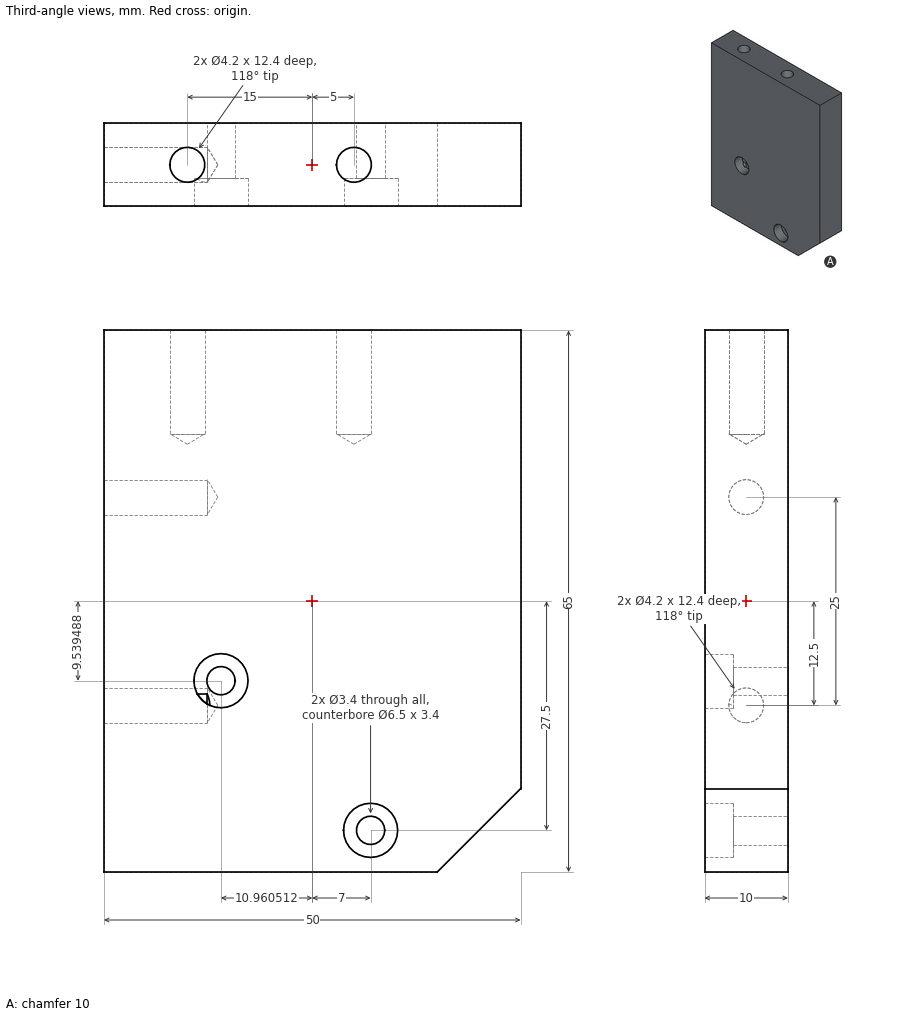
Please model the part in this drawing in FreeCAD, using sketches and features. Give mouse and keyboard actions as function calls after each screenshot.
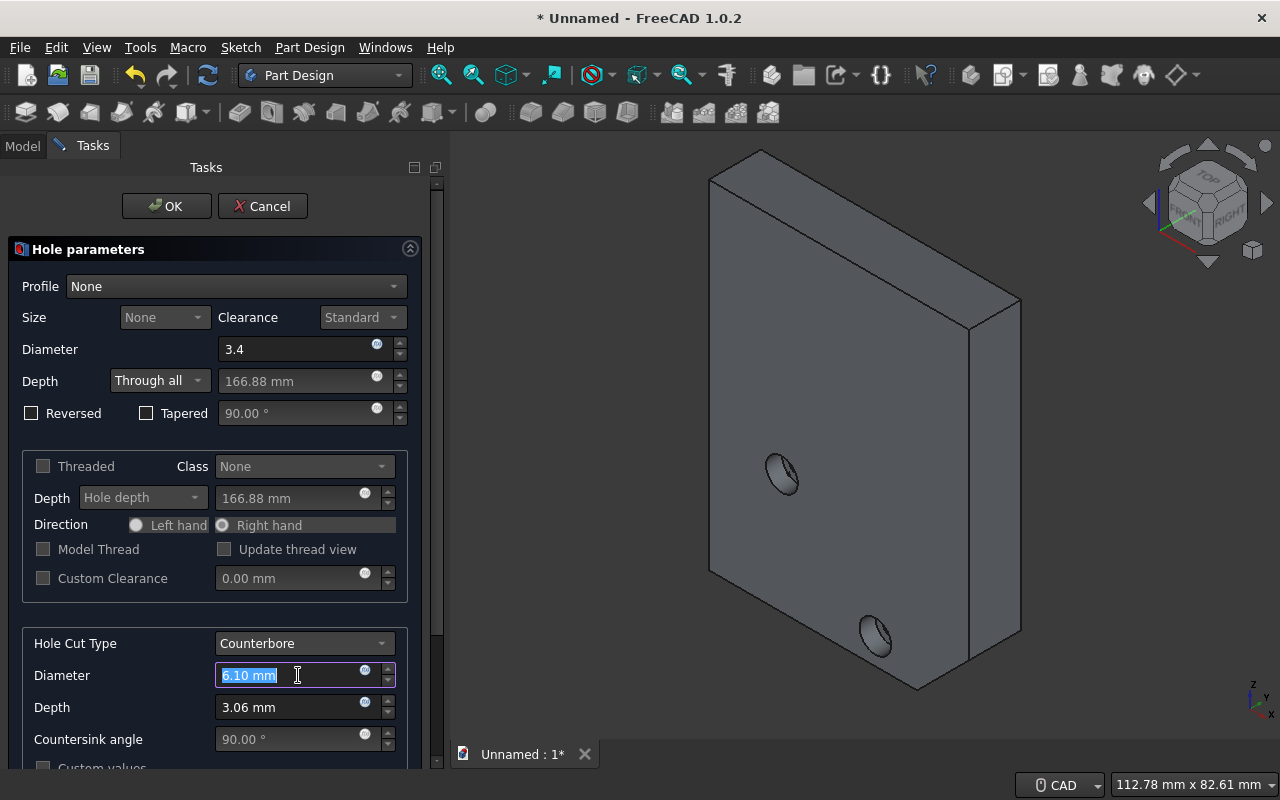
text(6.5)
key(Tab)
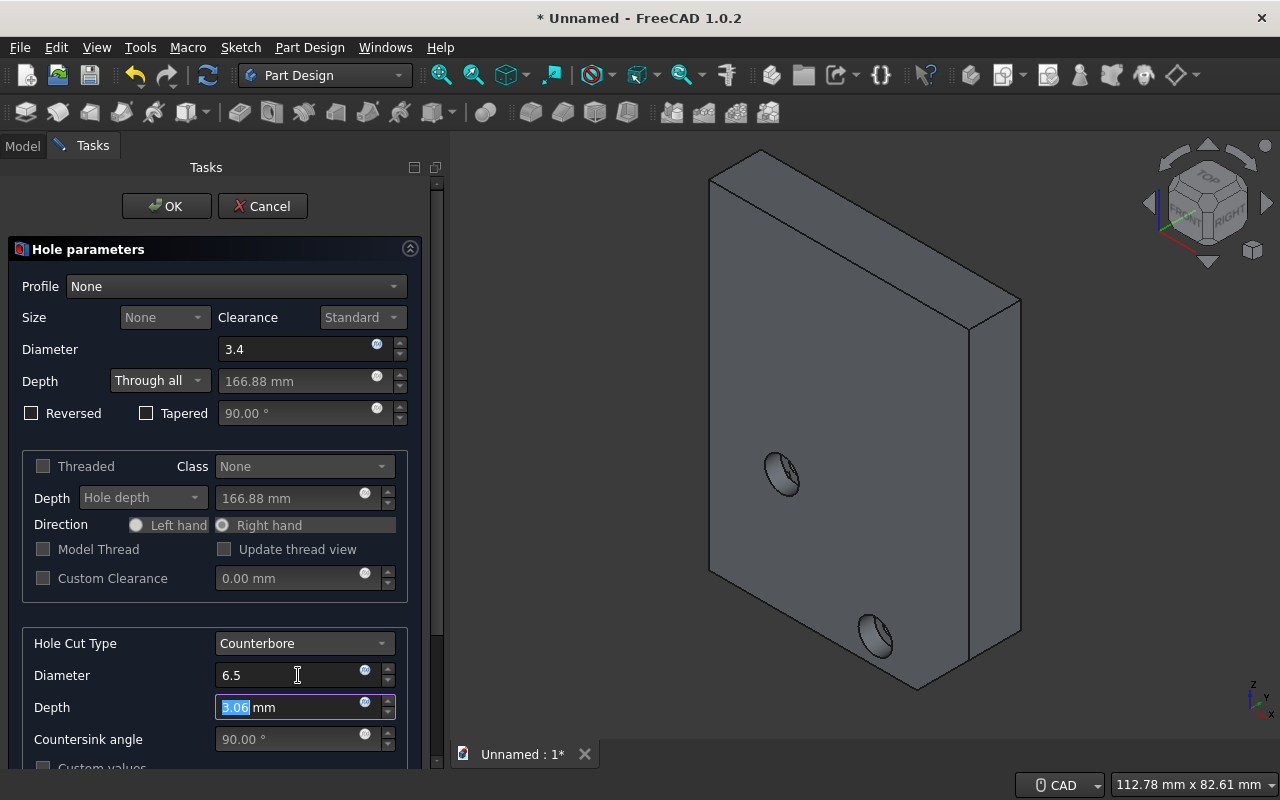
text(3.4)
key(Tab)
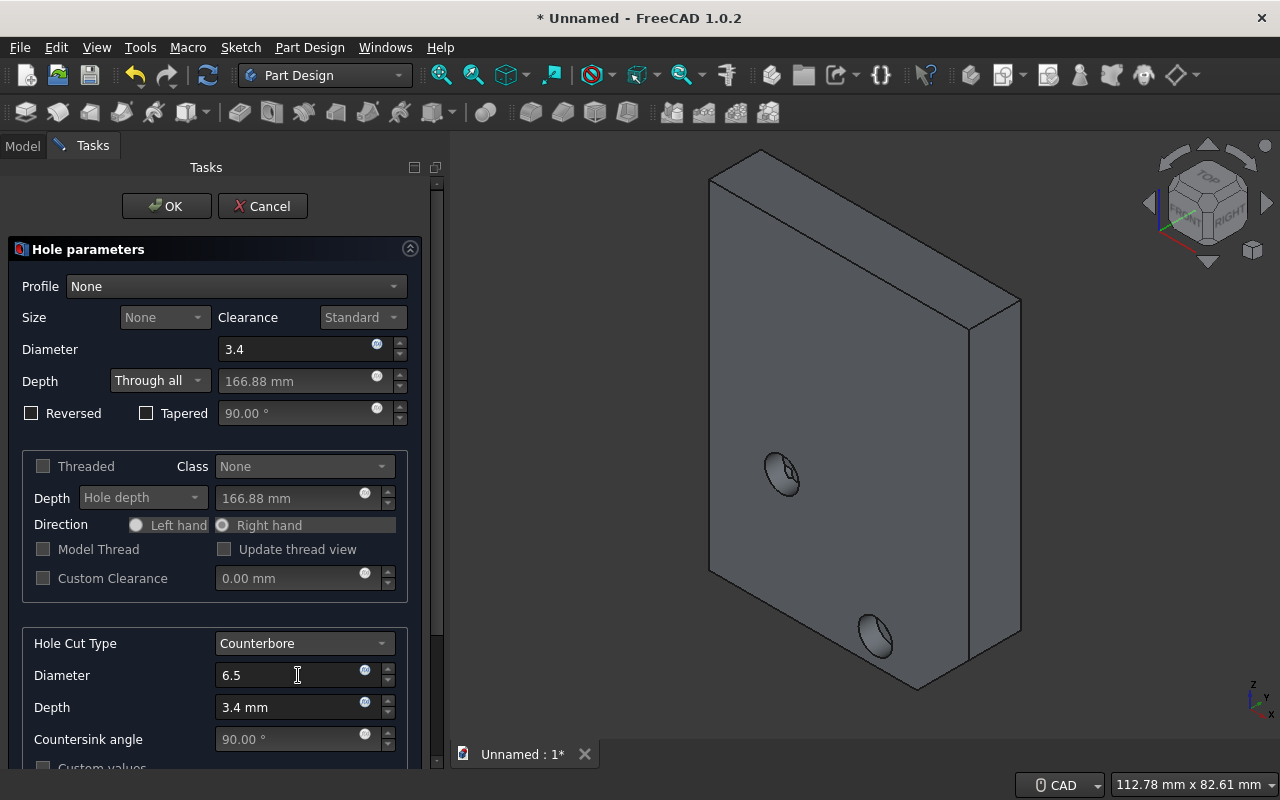
click(167, 206)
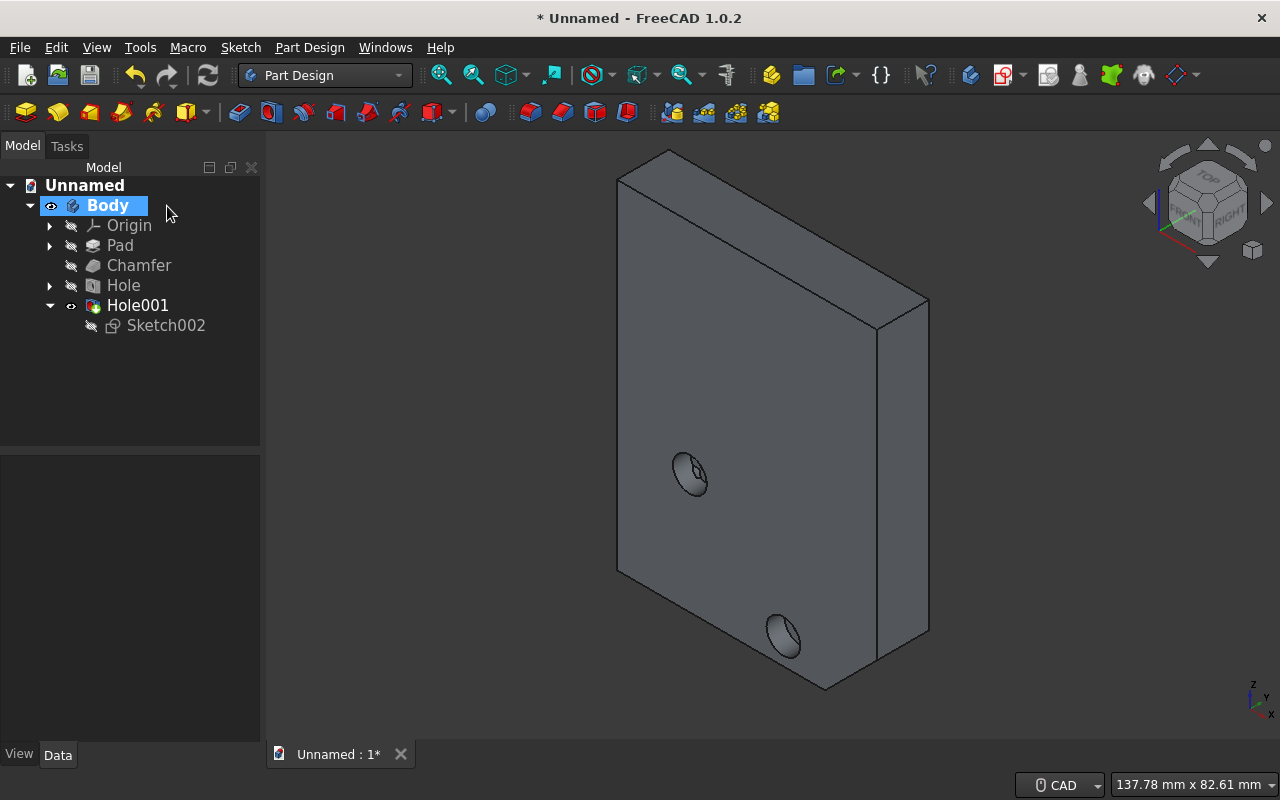
click(847, 282)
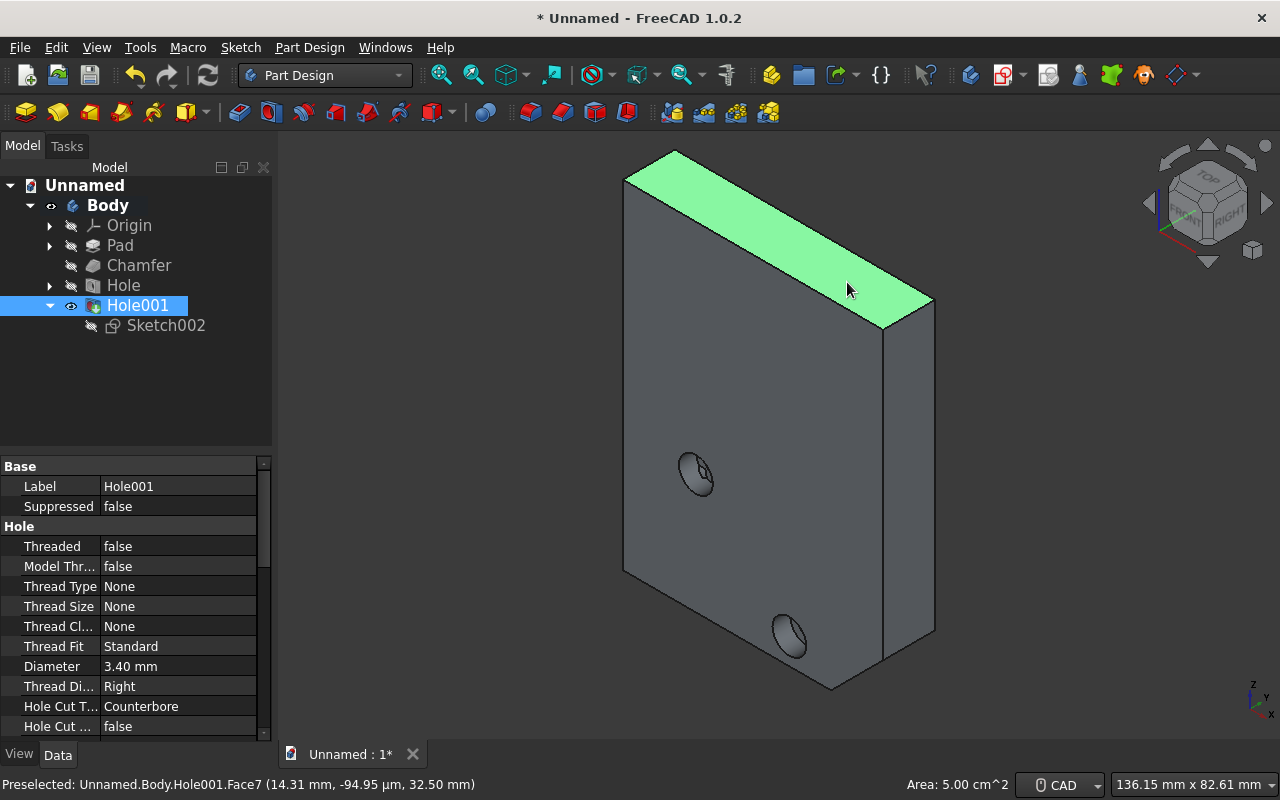
click(1004, 76)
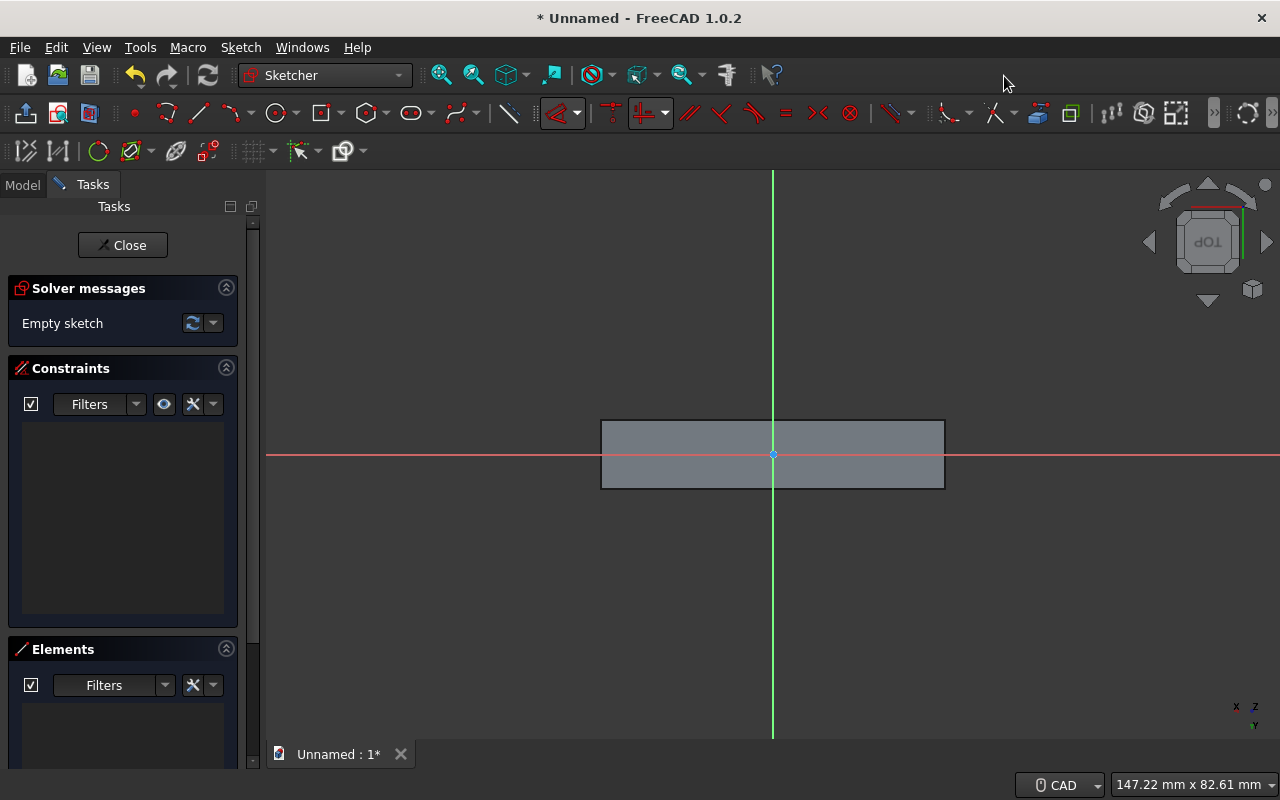
scroll(852, 455, up, 6)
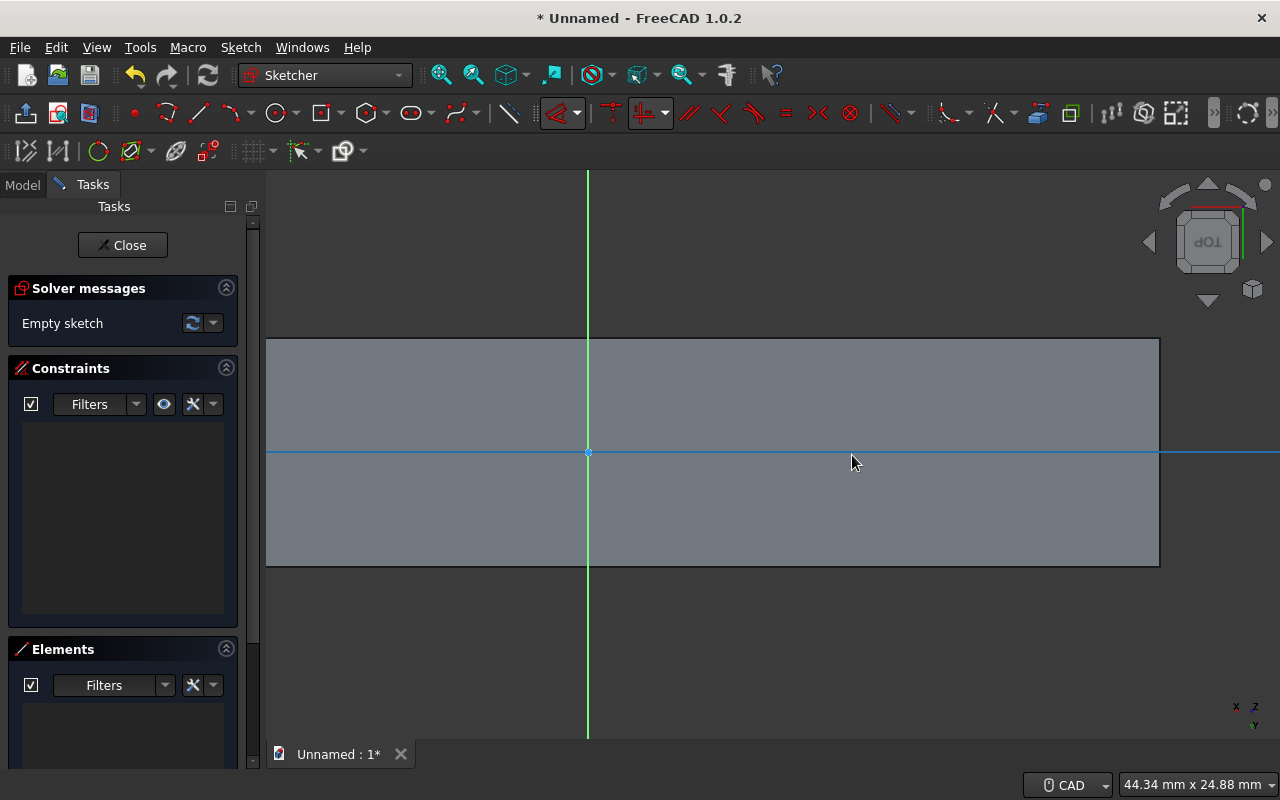
key(g)
key(c)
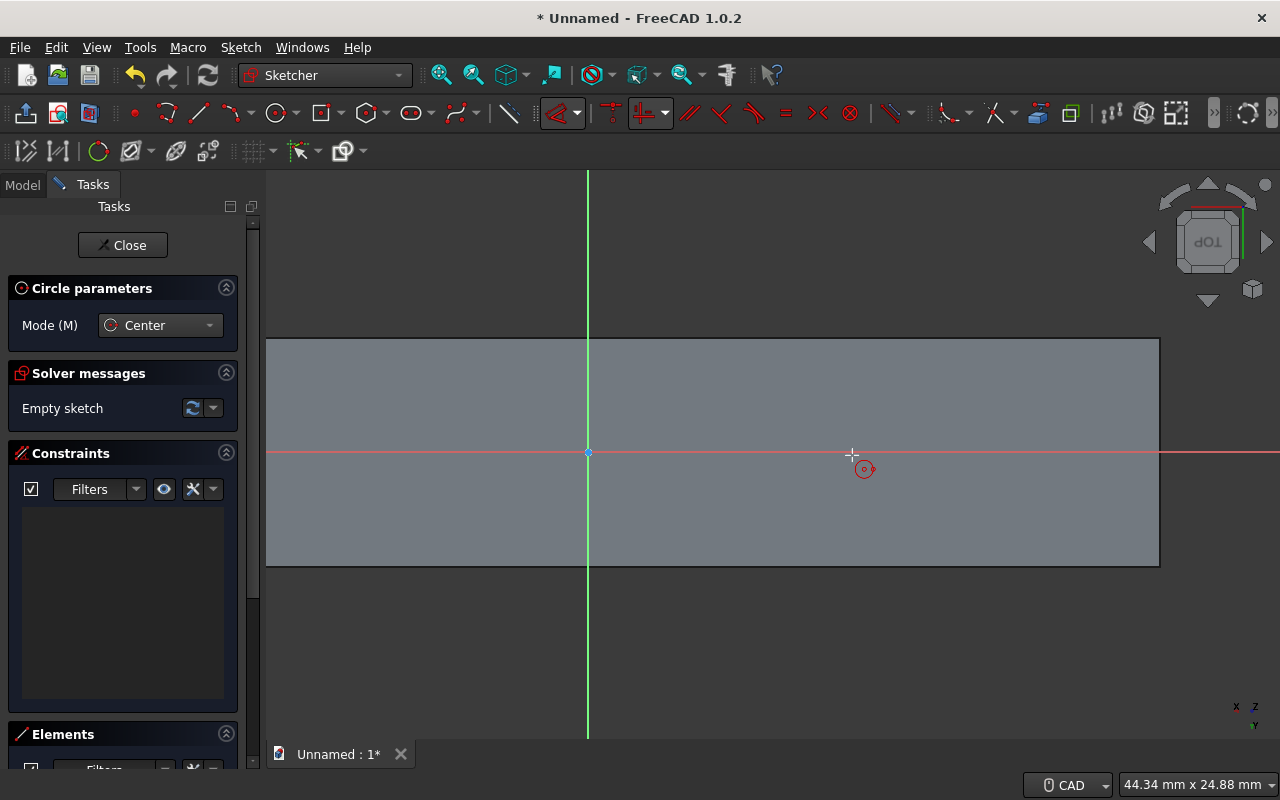
click(931, 452)
move(965, 418)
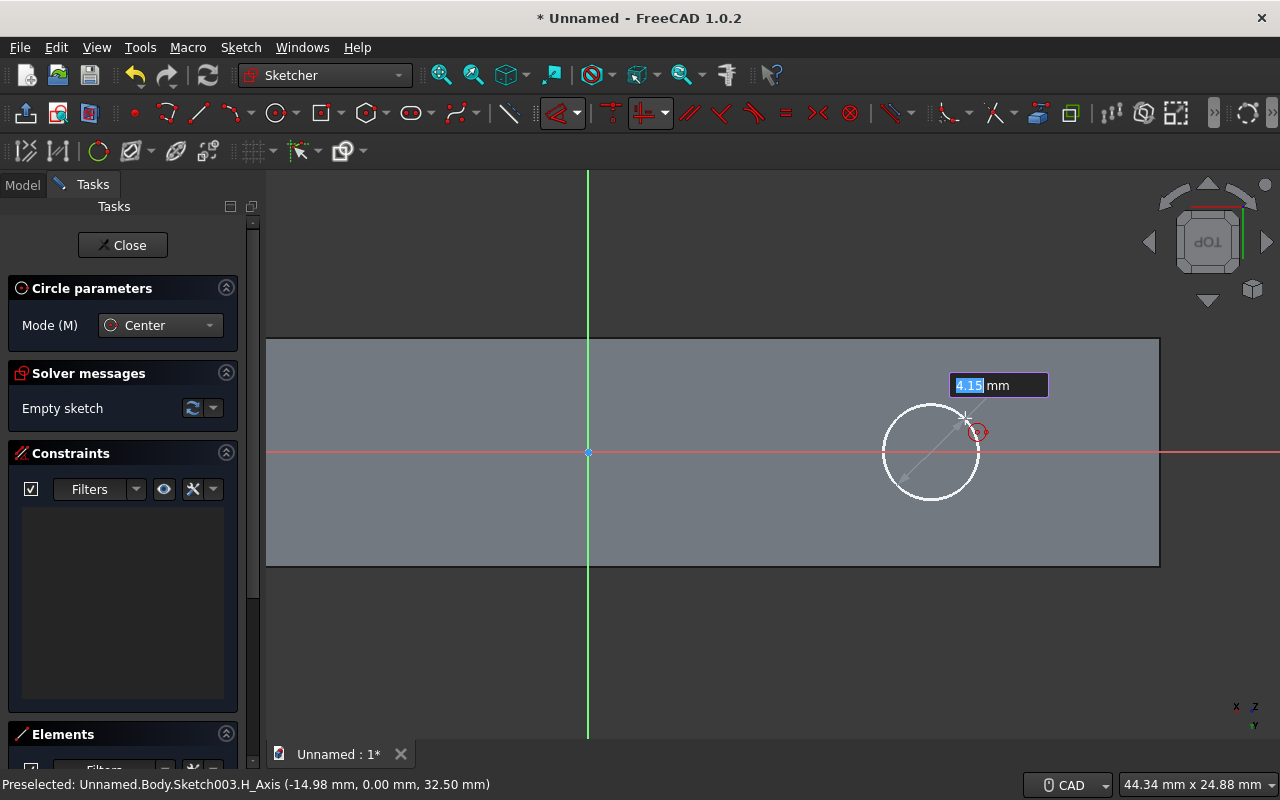
text(4.2)
key(Return)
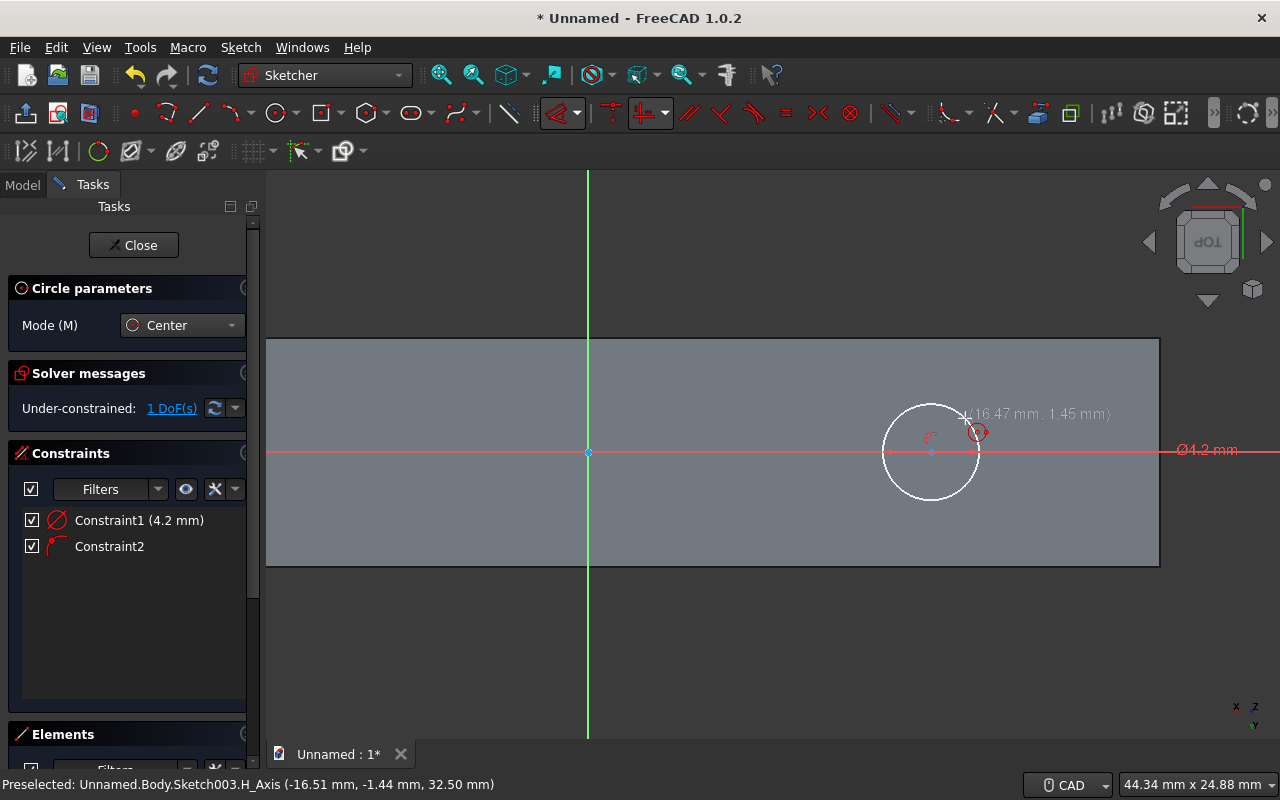
click(474, 452)
move(508, 418)